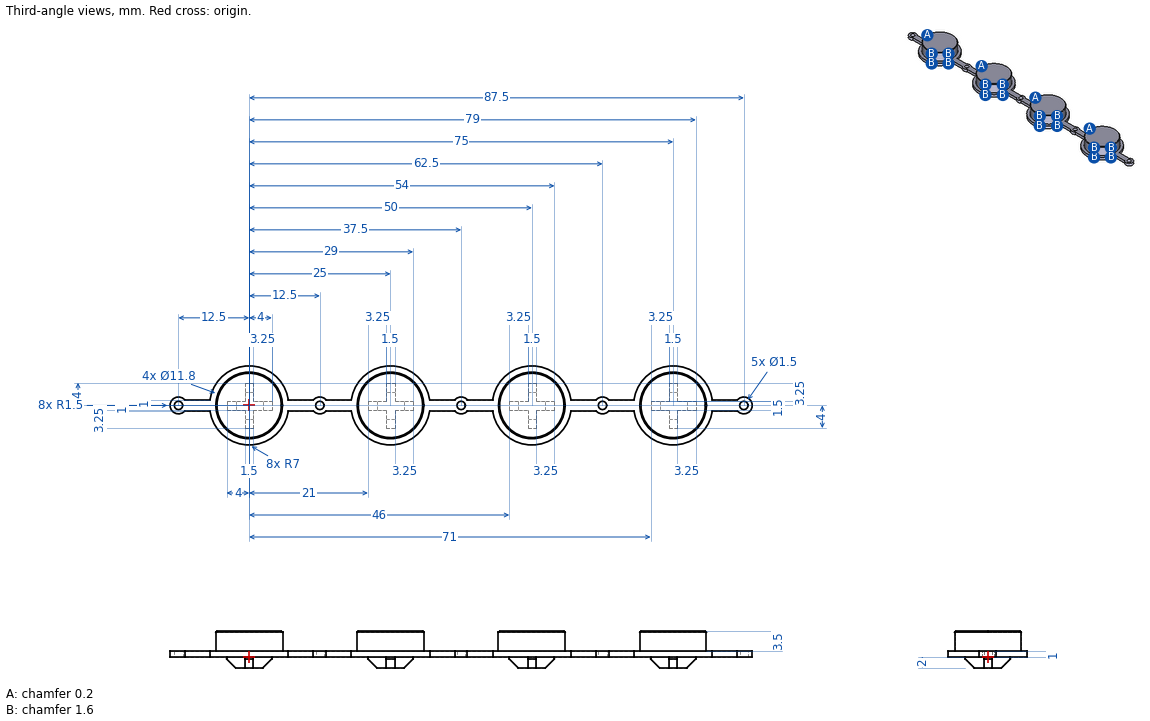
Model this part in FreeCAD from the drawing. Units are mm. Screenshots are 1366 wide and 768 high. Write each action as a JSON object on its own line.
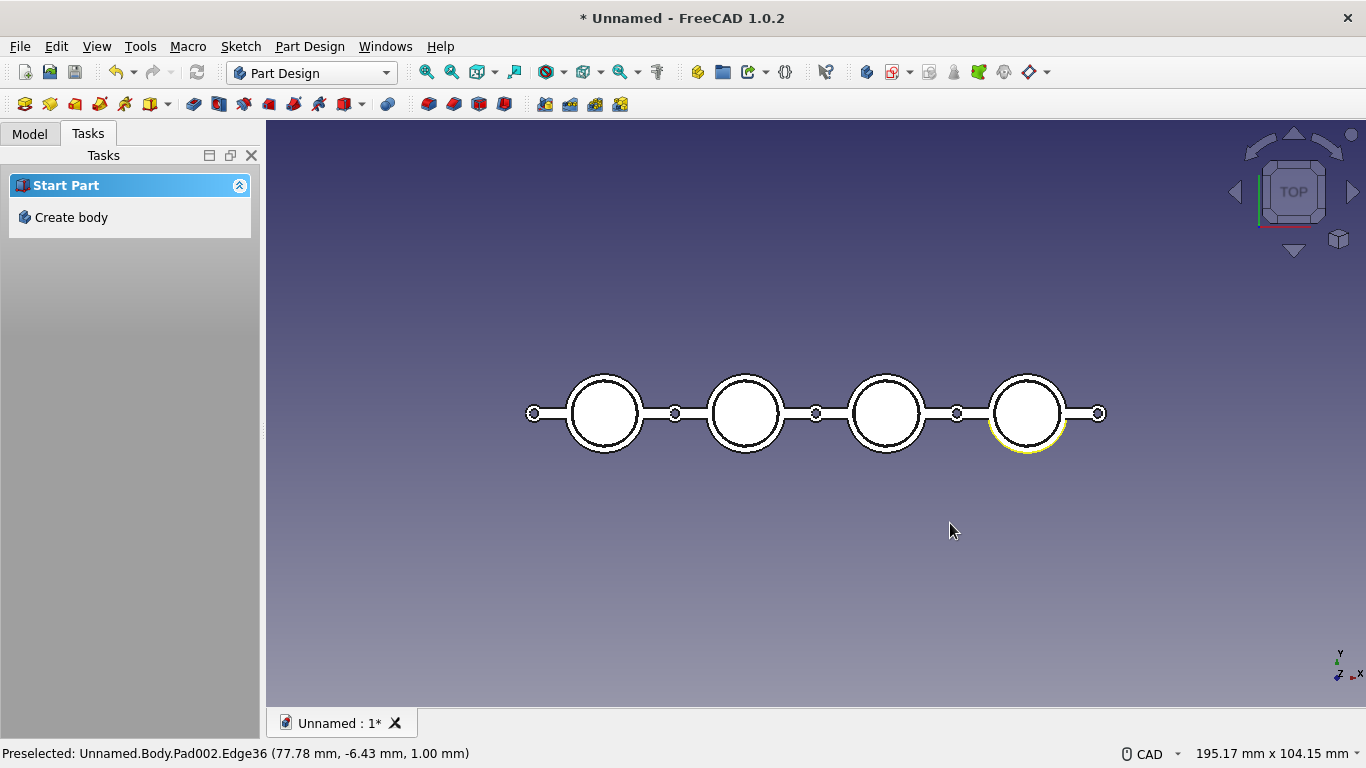
{"action": "scroll", "coordinate": [1027, 435], "scroll_direction": "up", "scroll_amount": 8}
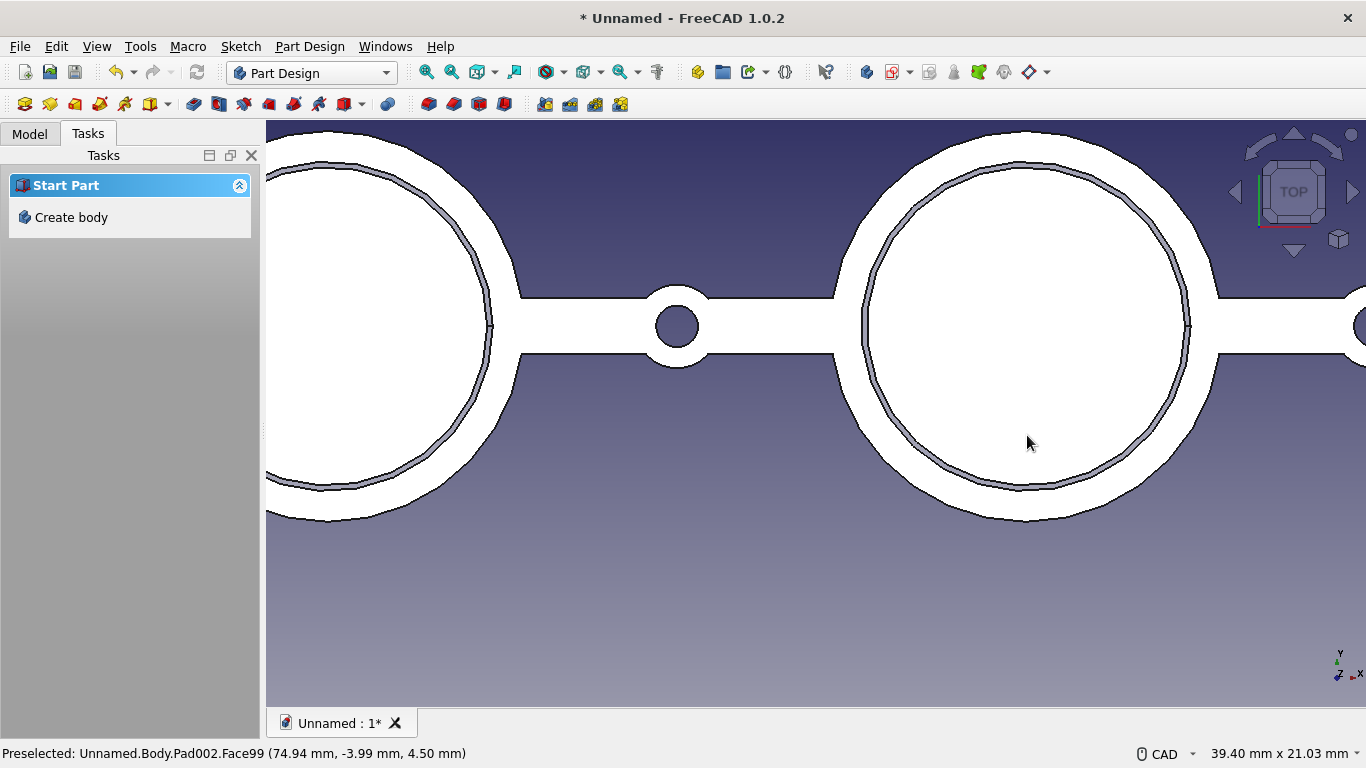
{"action": "left_click", "coordinate": [427, 72]}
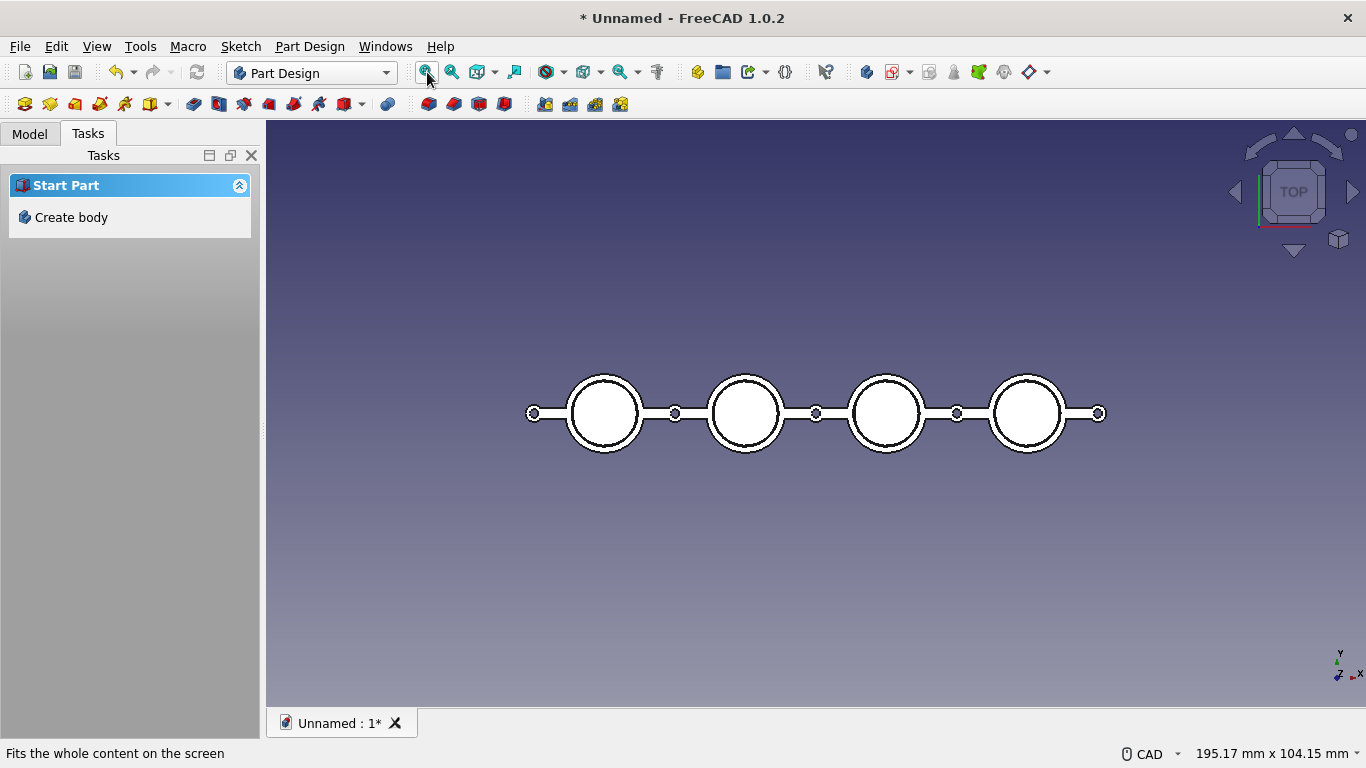
{"action": "key", "text": "1"}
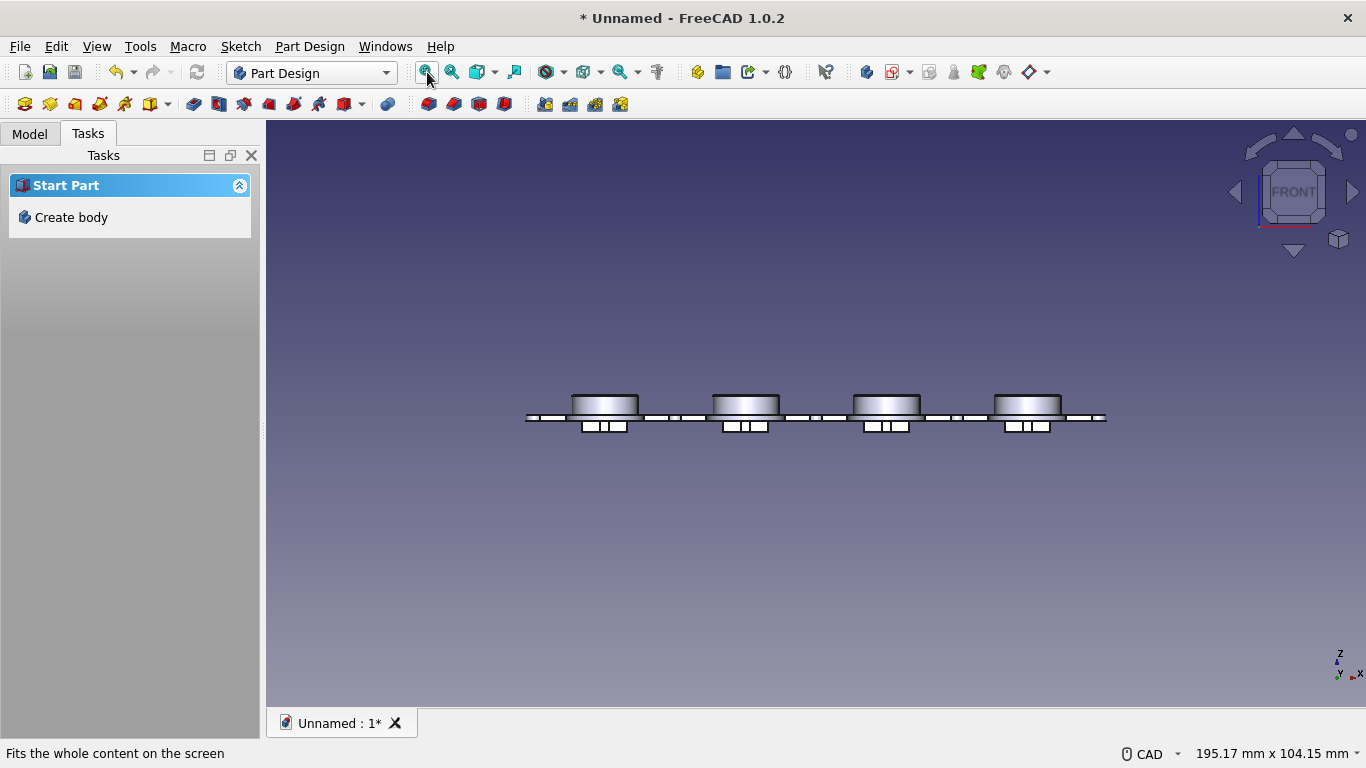
{"action": "scroll", "coordinate": [1027, 431], "scroll_direction": "up", "scroll_amount": 8}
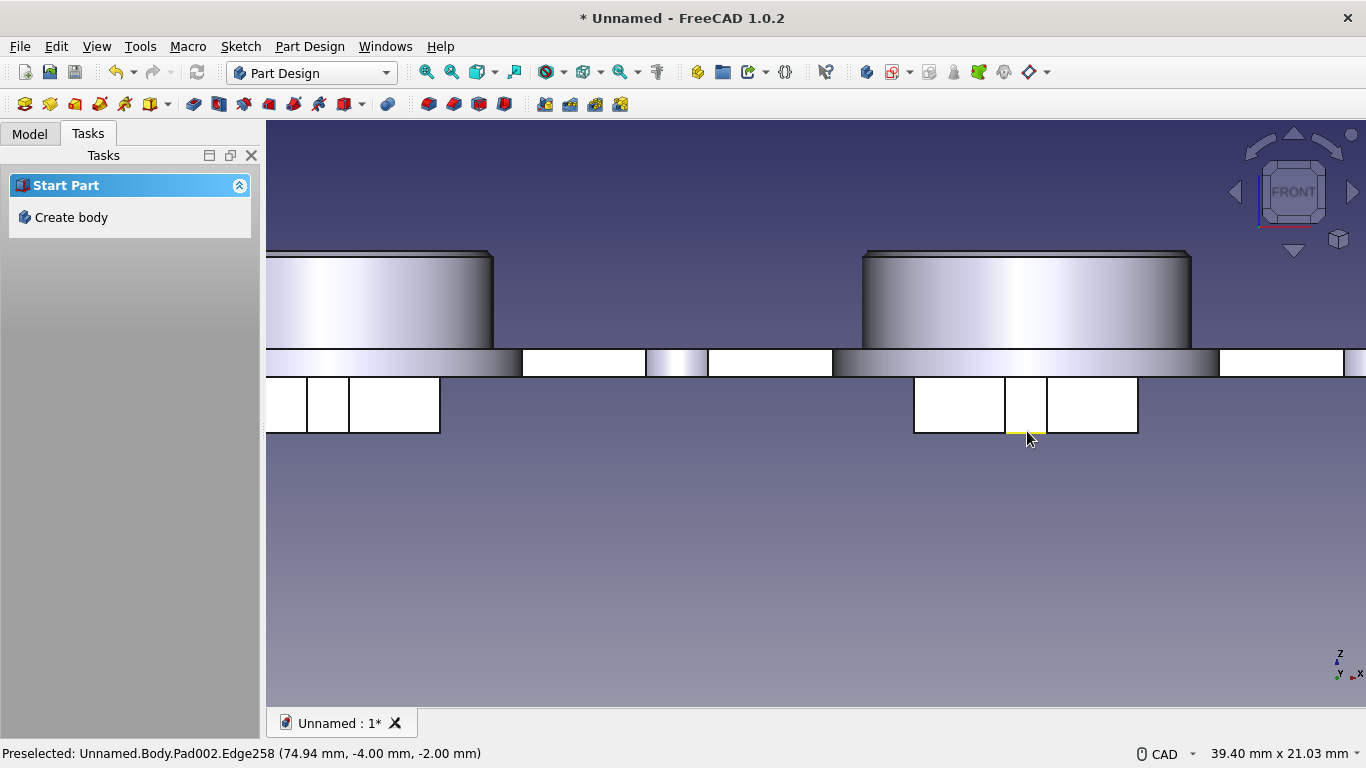
{"action": "left_click", "coordinate": [1026, 432]}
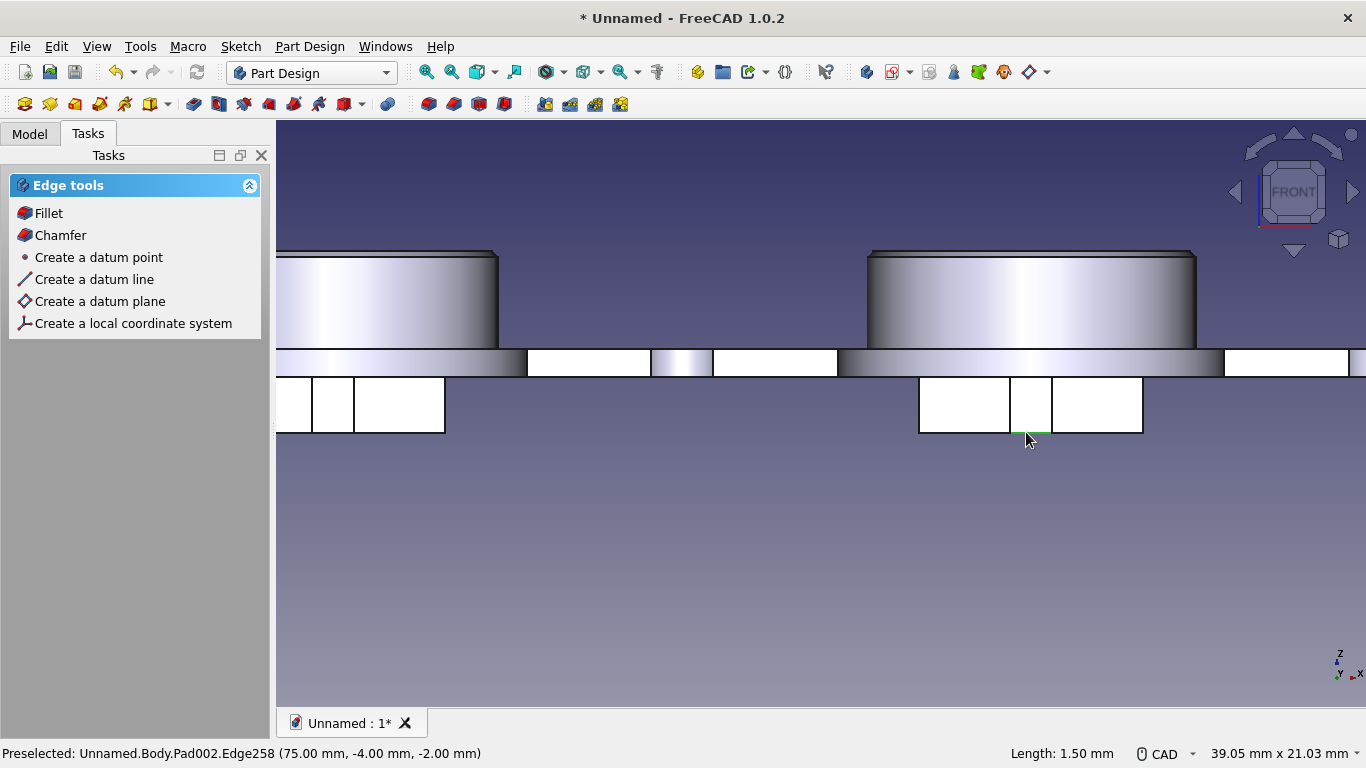
{"action": "left_click", "coordinate": [333, 432], "text": "ctrl"}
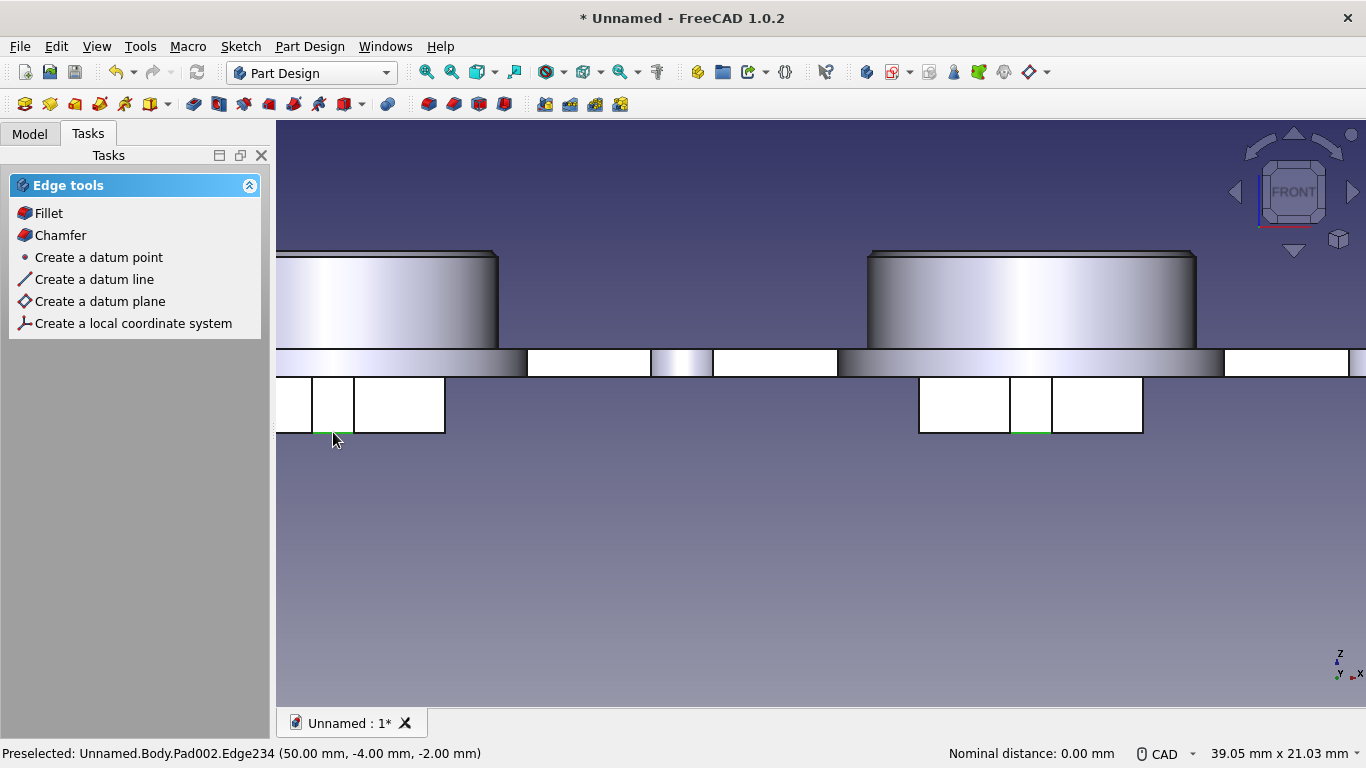
{"action": "key", "text": "v f"}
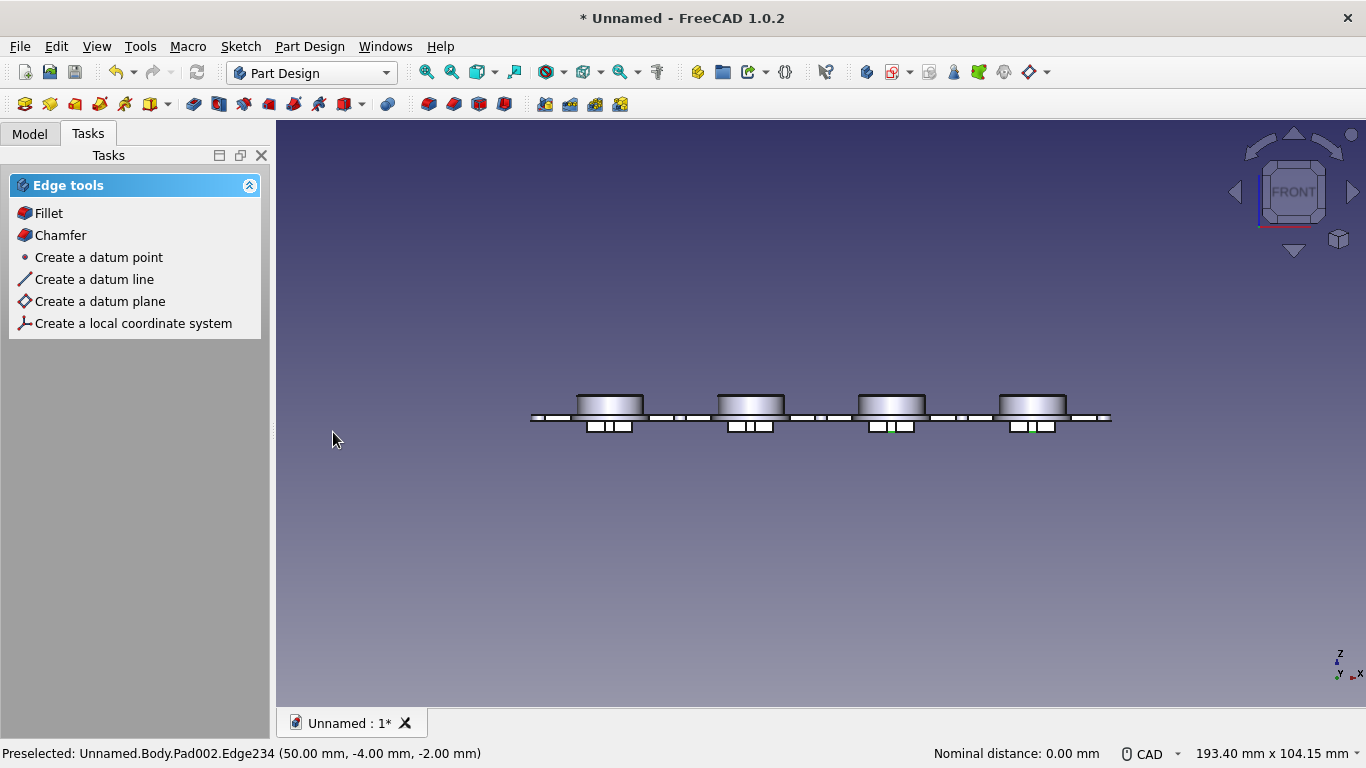
{"action": "key", "text": "3"}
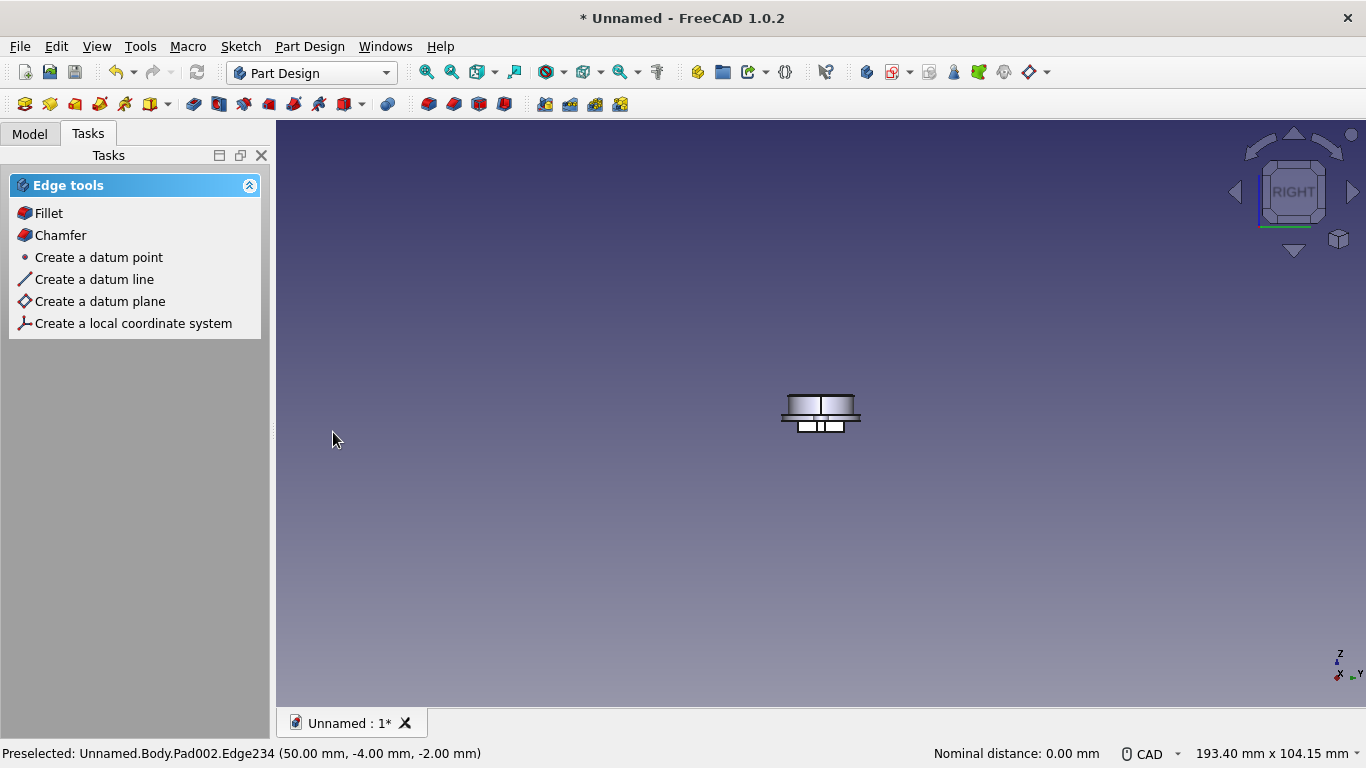
{"action": "left_click", "coordinate": [427, 72]}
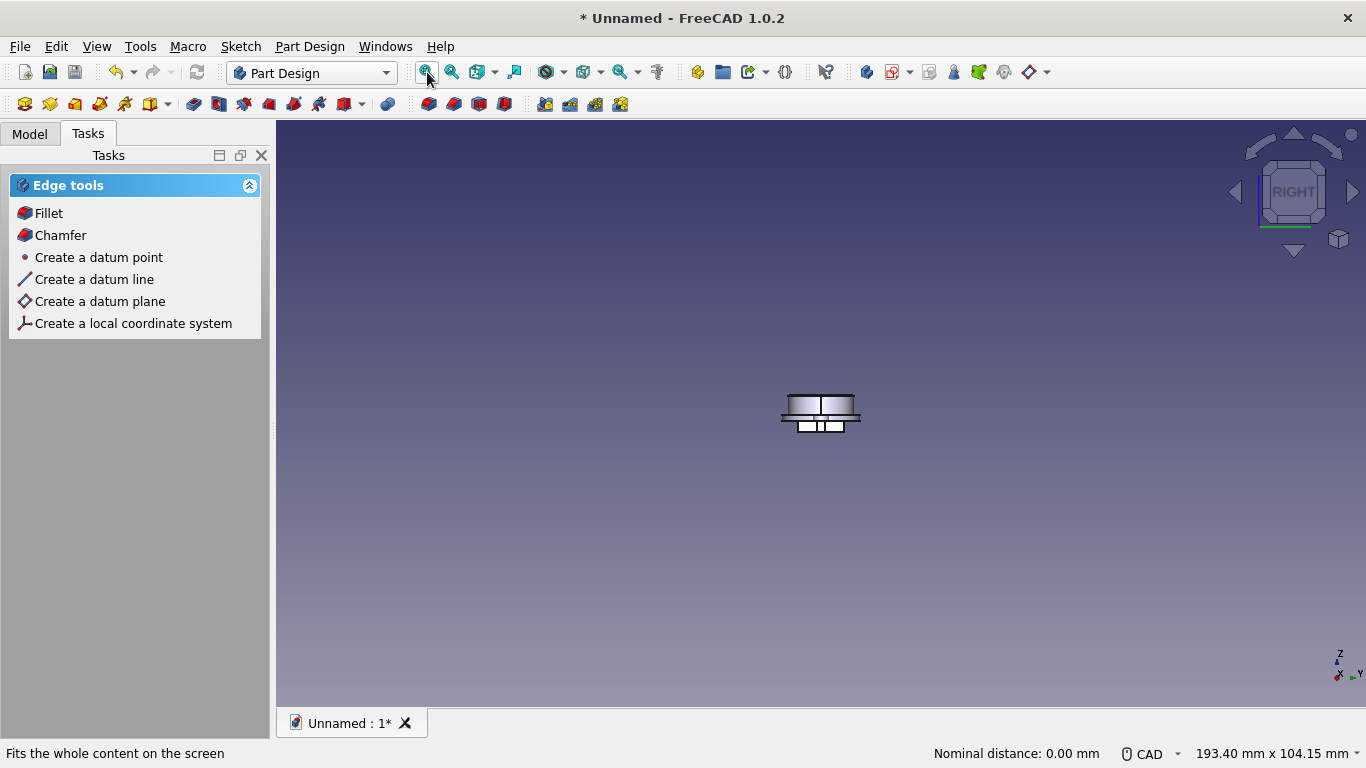
{"action": "scroll", "coordinate": [821, 431], "scroll_direction": "up", "scroll_amount": 8}